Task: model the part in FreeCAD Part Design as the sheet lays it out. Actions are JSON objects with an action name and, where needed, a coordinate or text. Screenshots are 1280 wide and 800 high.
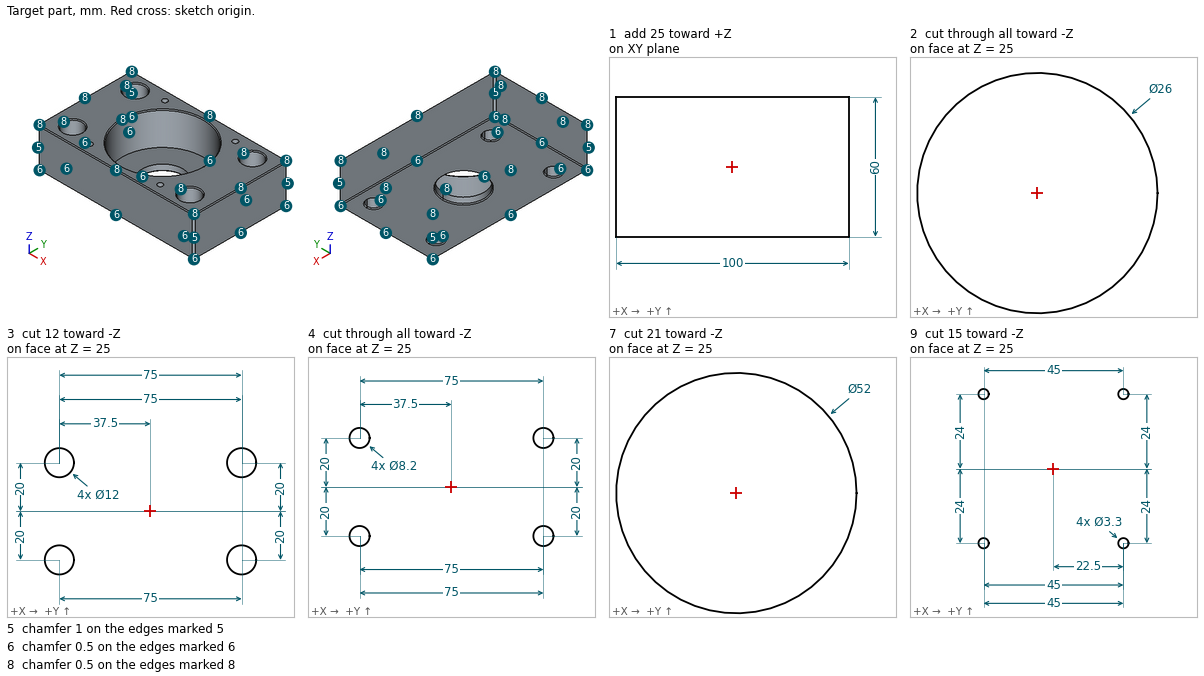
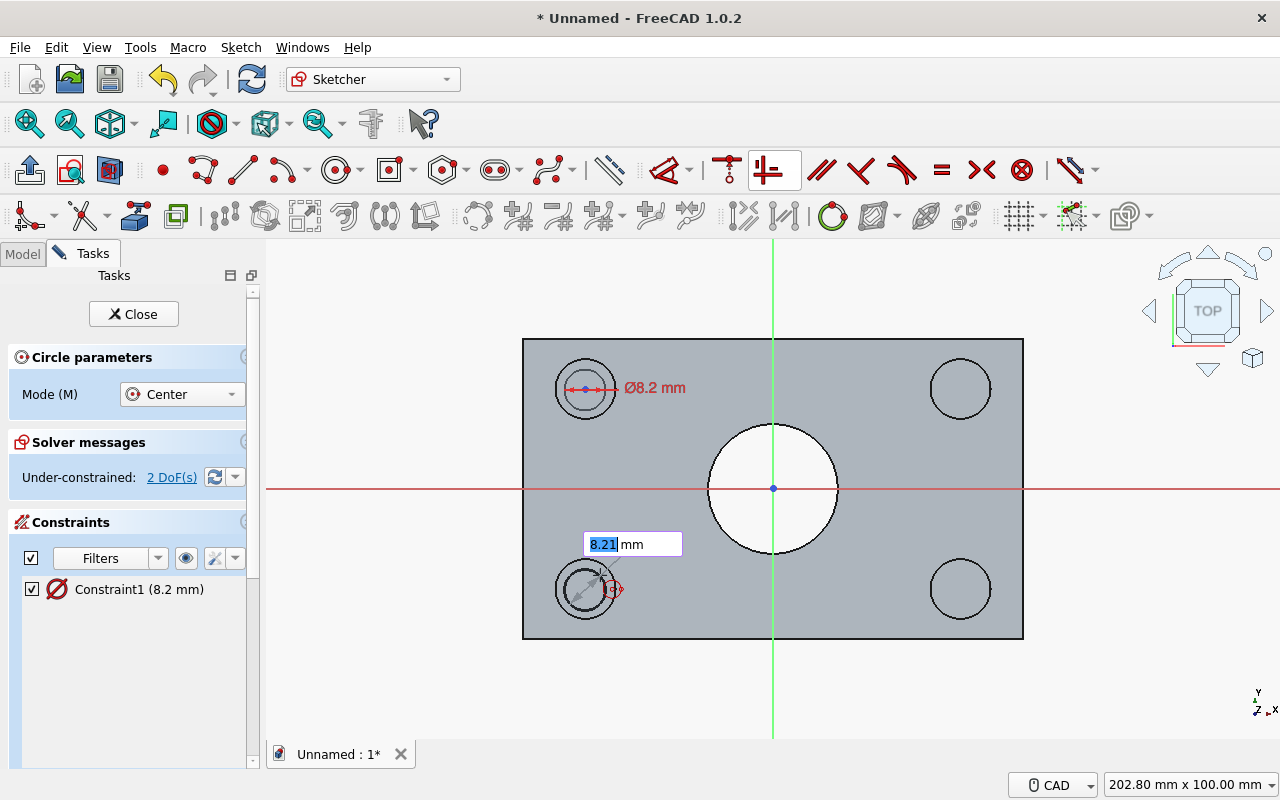
{"action": "type", "text": "8.2"}
{"action": "key", "text": "Return"}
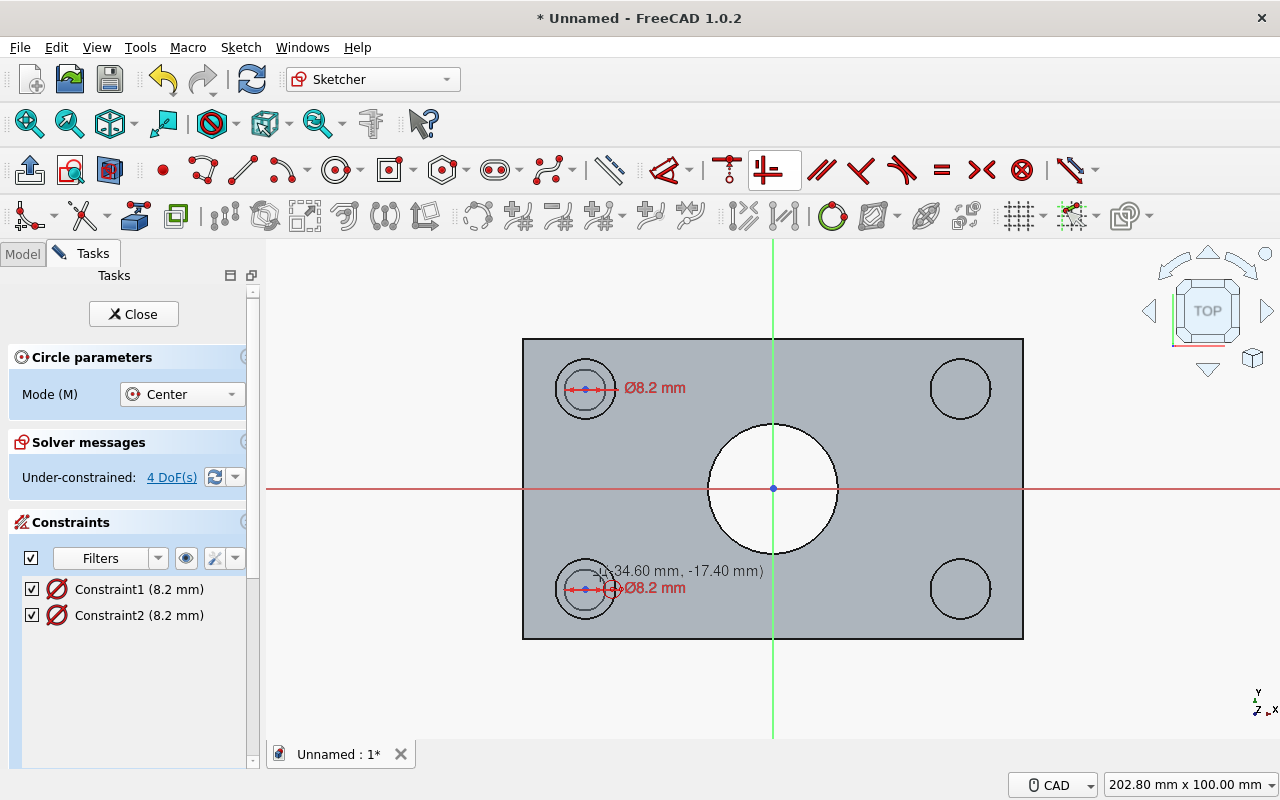
{"action": "left_click", "coordinate": [960, 389]}
{"action": "mouse_move", "coordinate": [975, 375]}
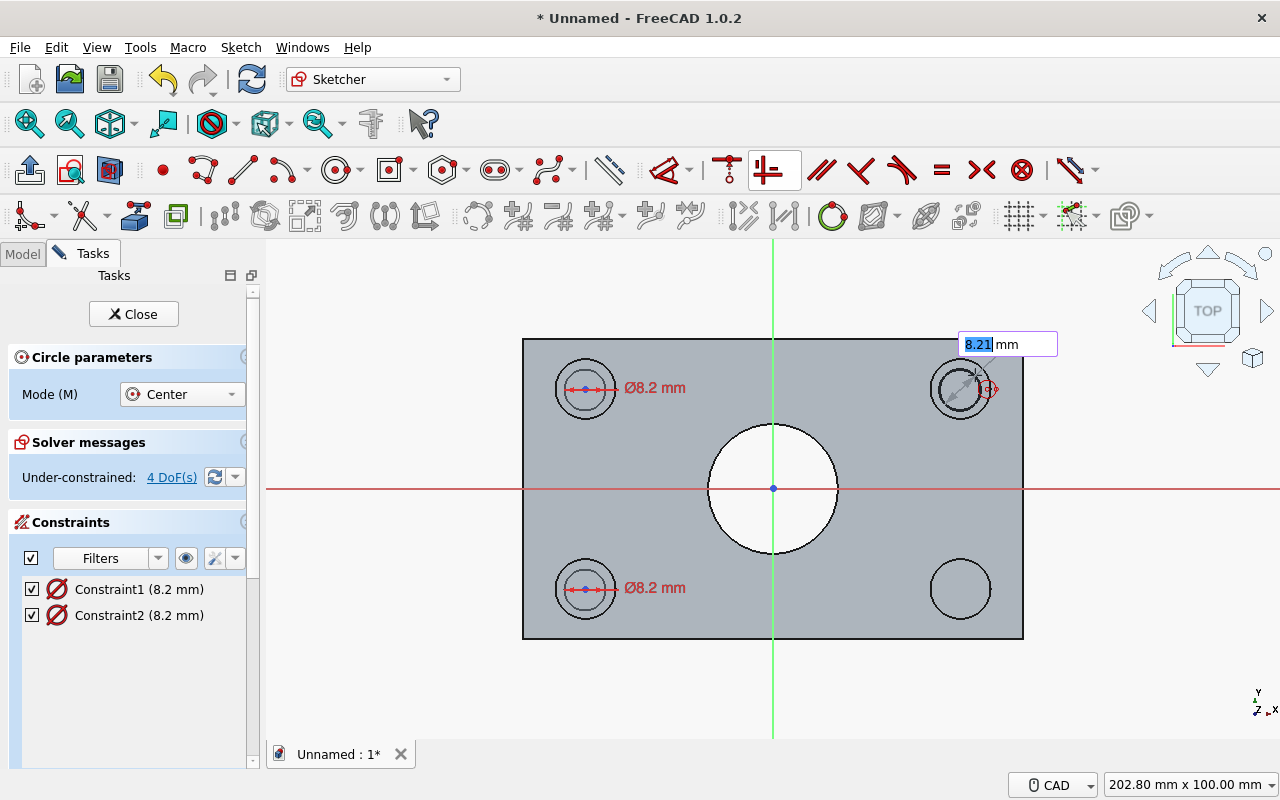
{"action": "type", "text": "8.2"}
{"action": "key", "text": "Return"}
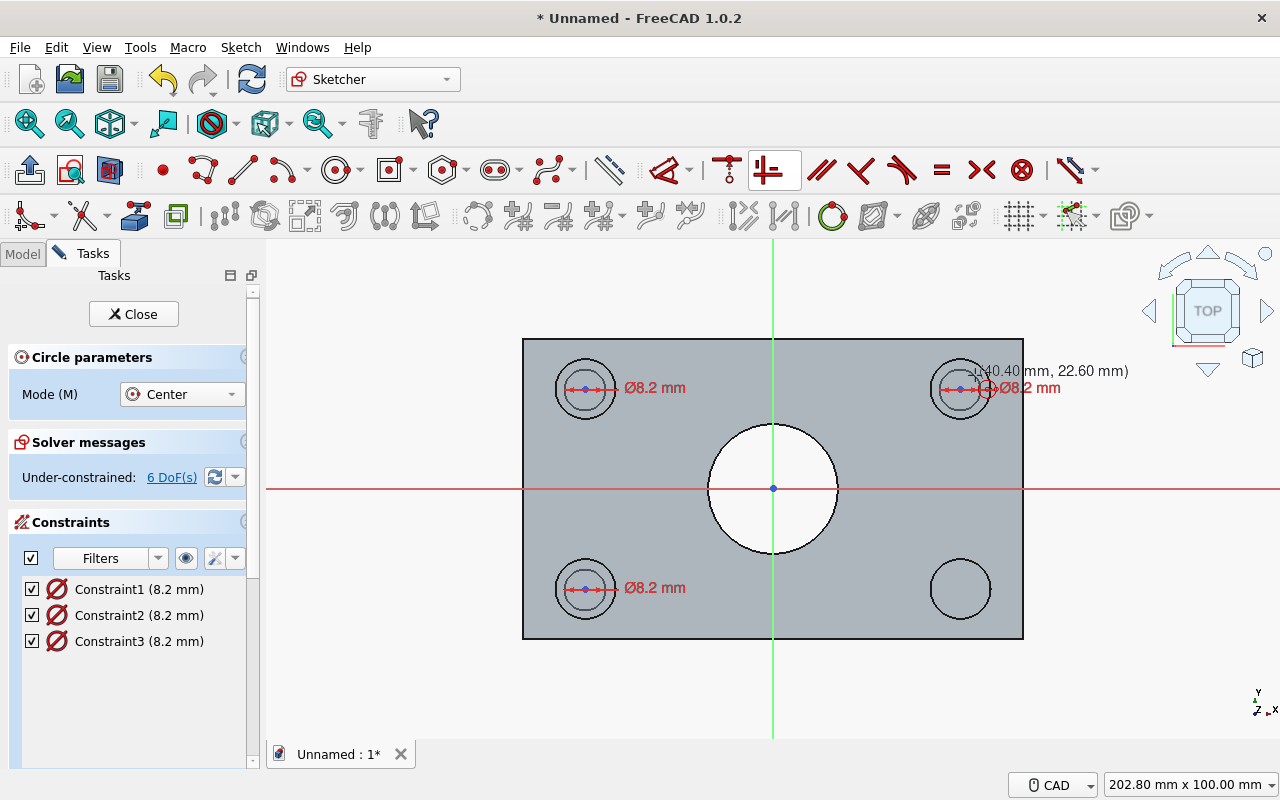
{"action": "left_click", "coordinate": [960, 589]}
{"action": "mouse_move", "coordinate": [975, 575]}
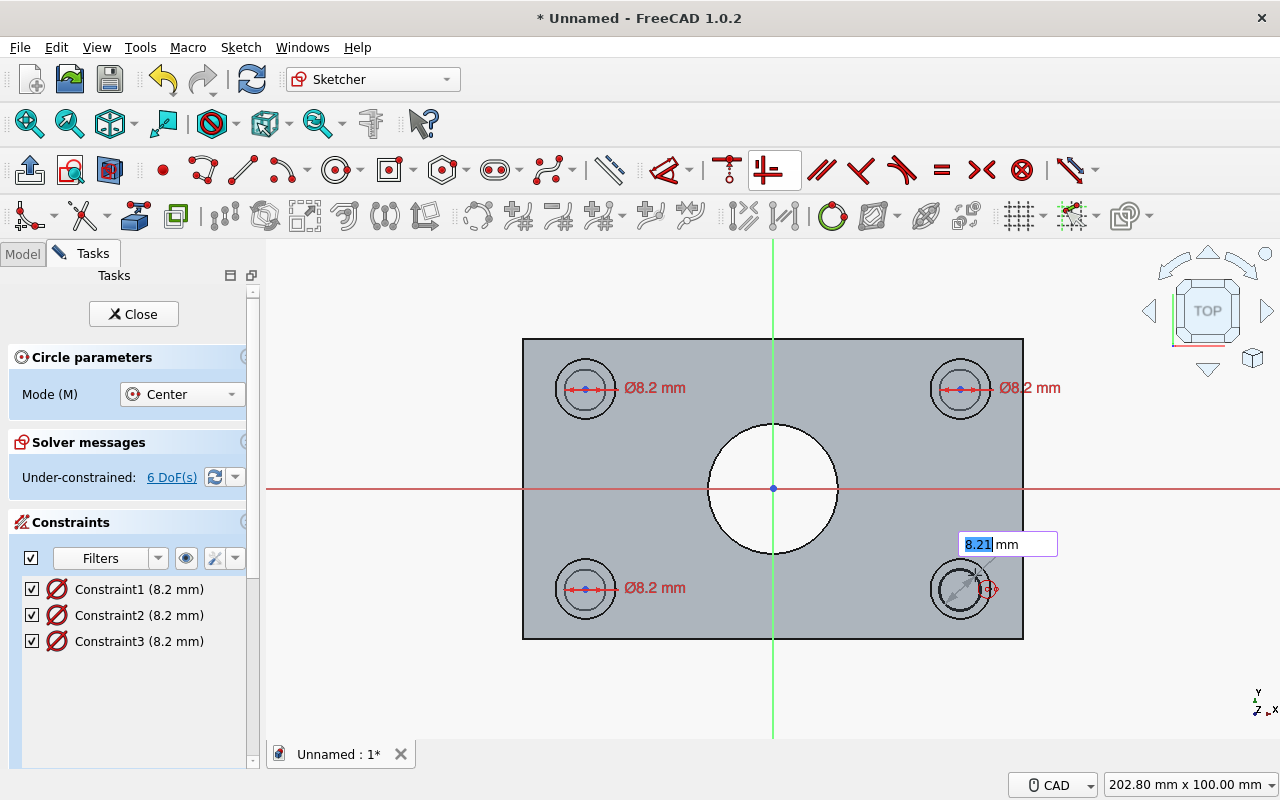
{"action": "type", "text": "8.2"}
{"action": "key", "text": "Return"}
{"action": "key", "text": "Escape"}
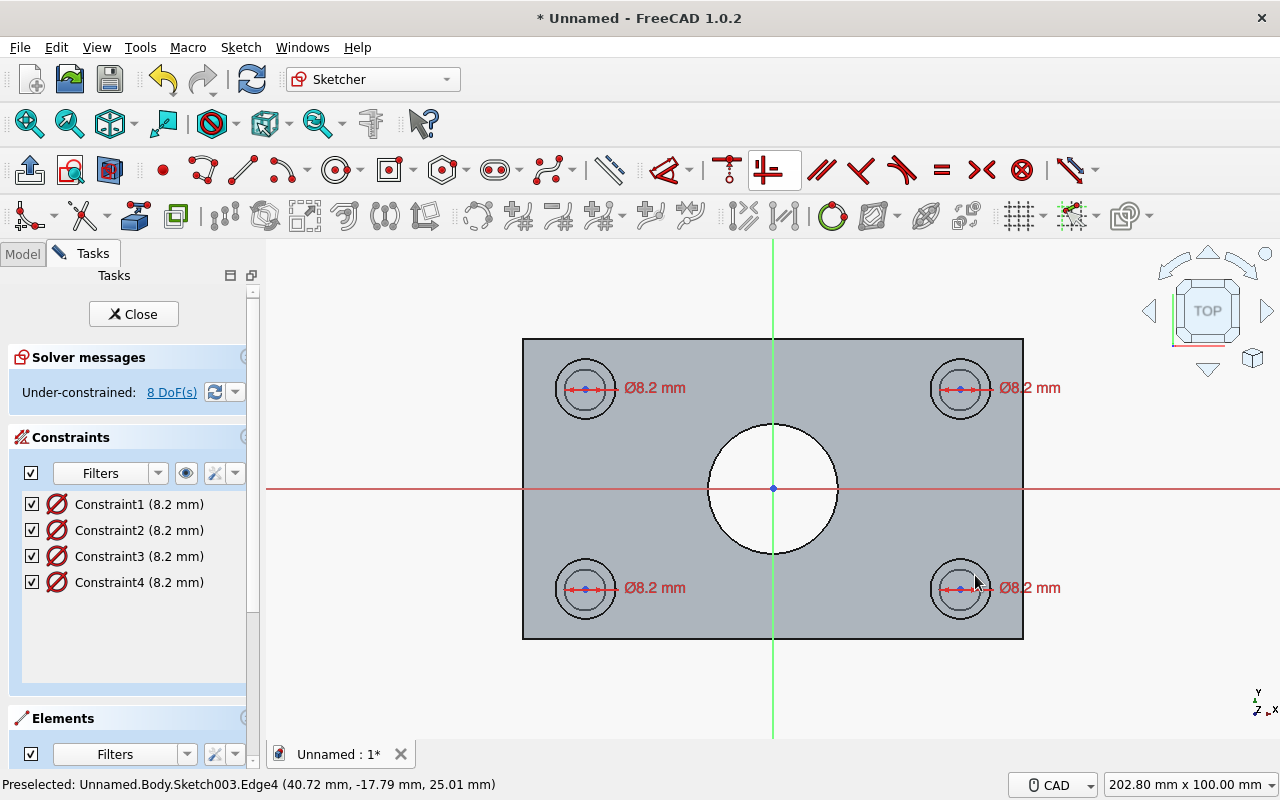
{"action": "left_click", "coordinate": [585, 390]}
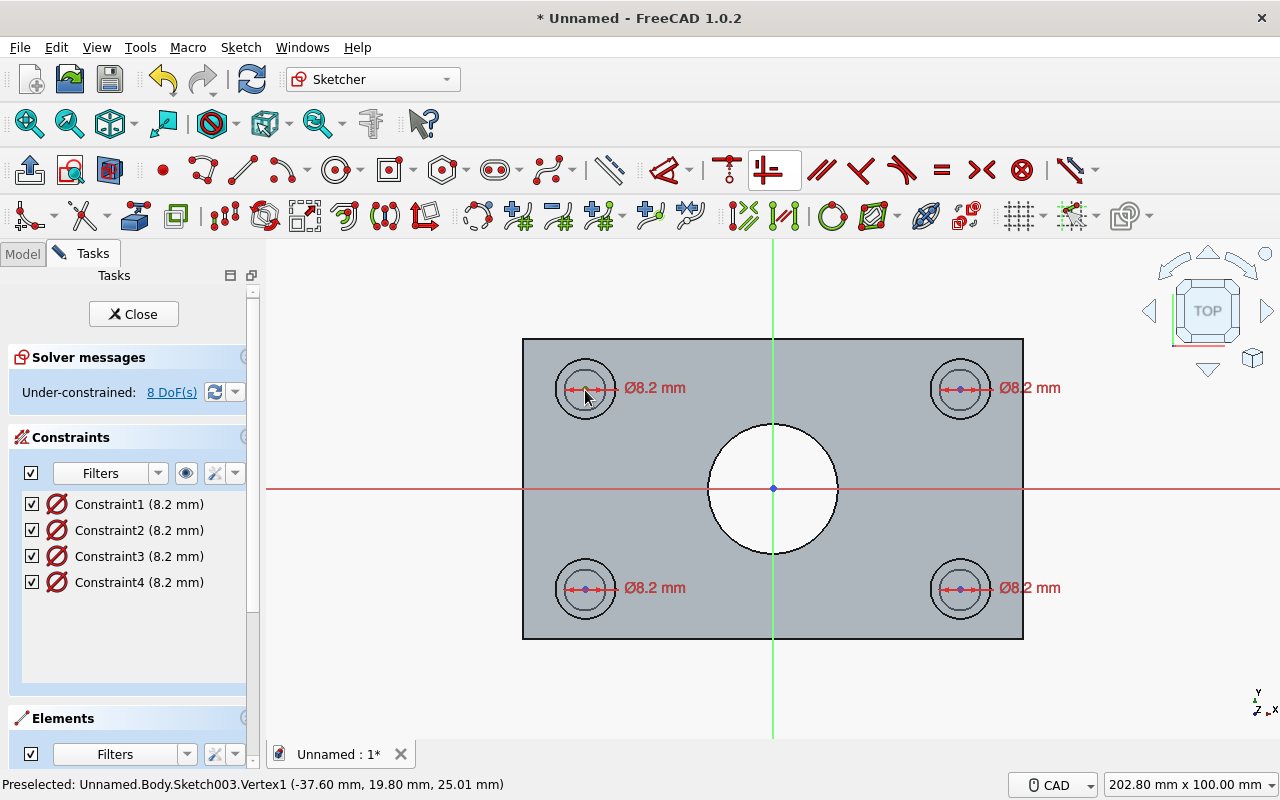
{"action": "key", "text": "i"}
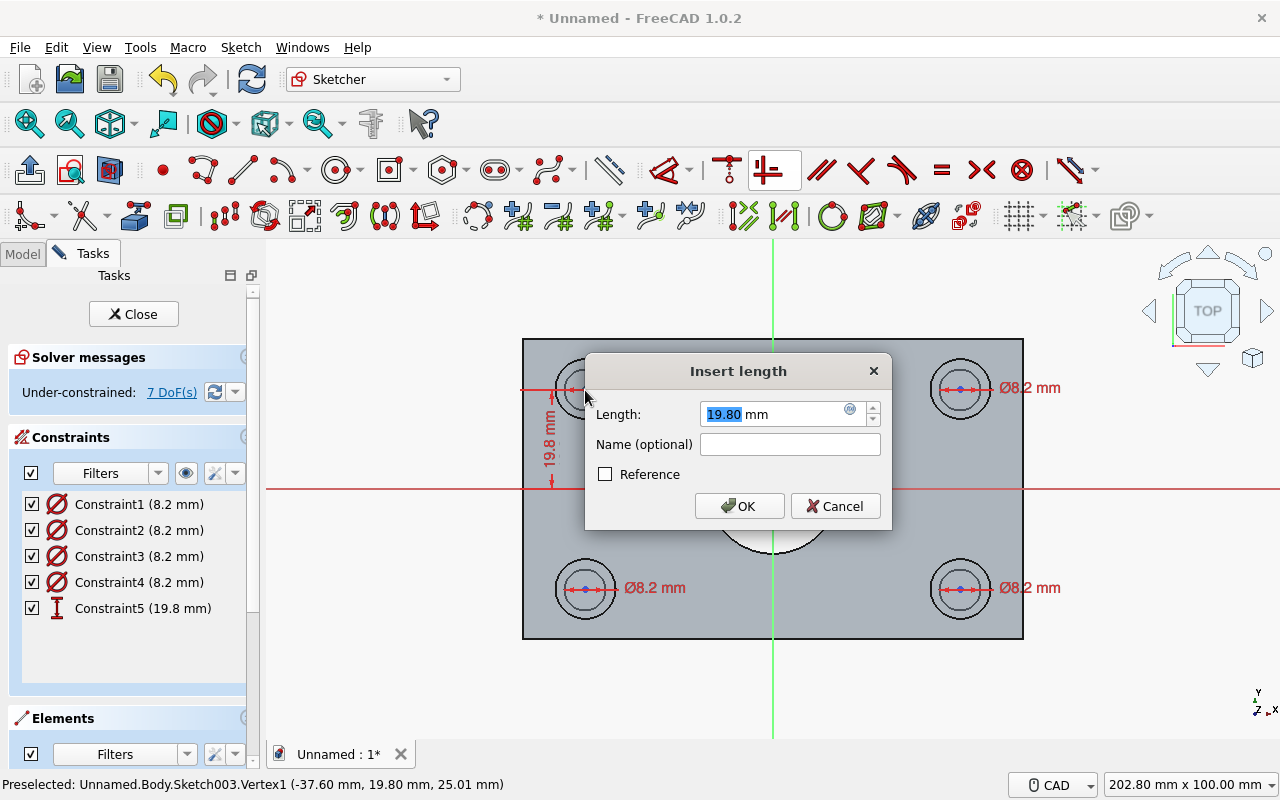
{"action": "type", "text": "20"}
{"action": "key", "text": "Return"}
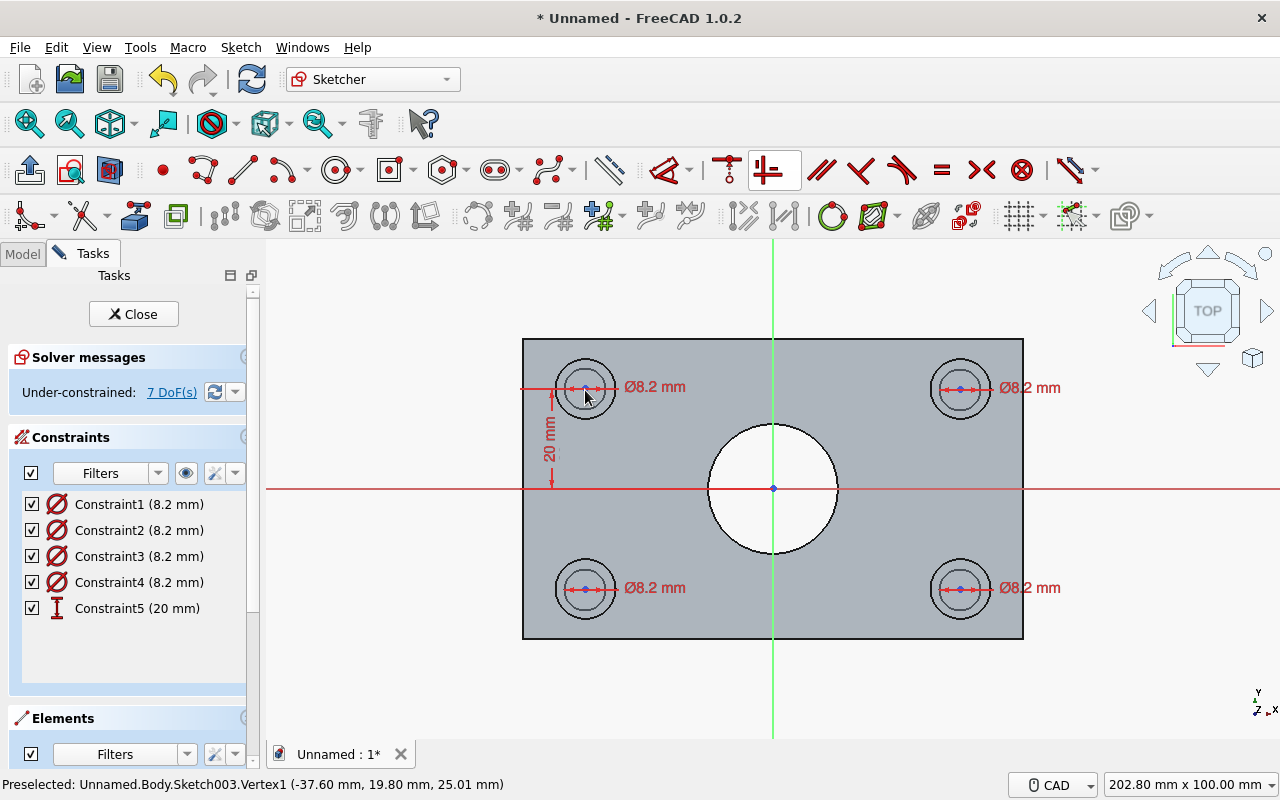
{"action": "left_click", "coordinate": [585, 590]}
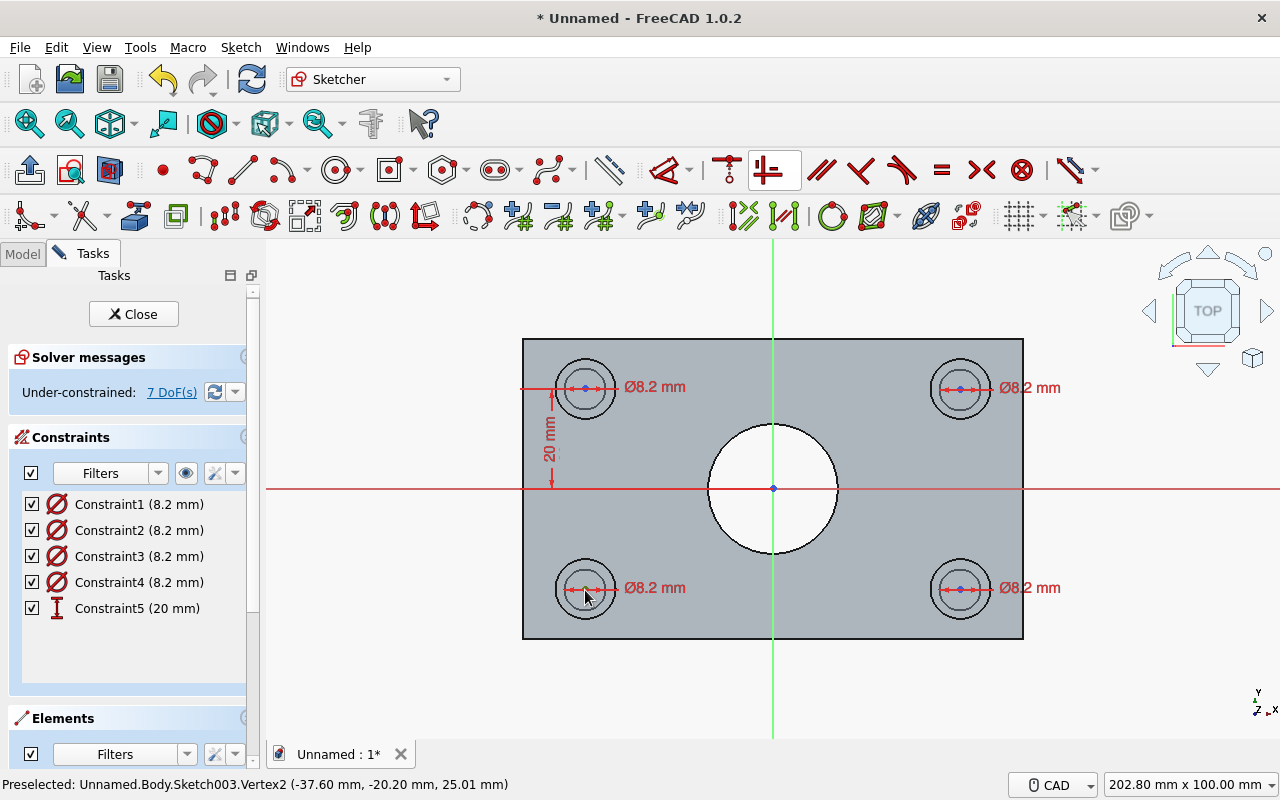
{"action": "key", "text": "i"}